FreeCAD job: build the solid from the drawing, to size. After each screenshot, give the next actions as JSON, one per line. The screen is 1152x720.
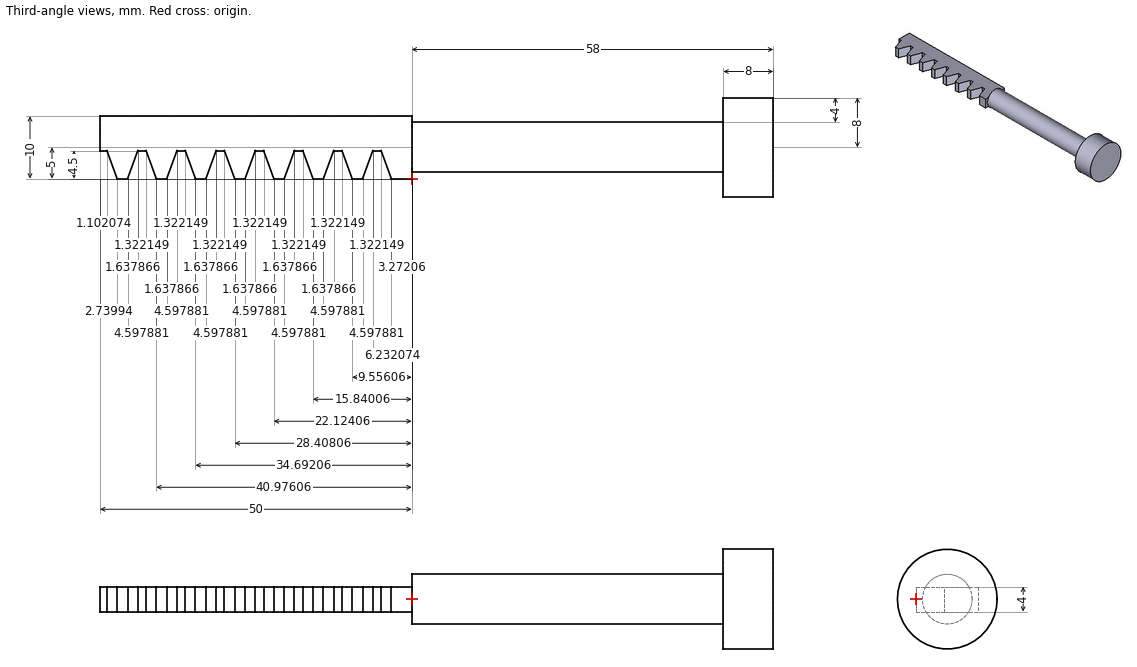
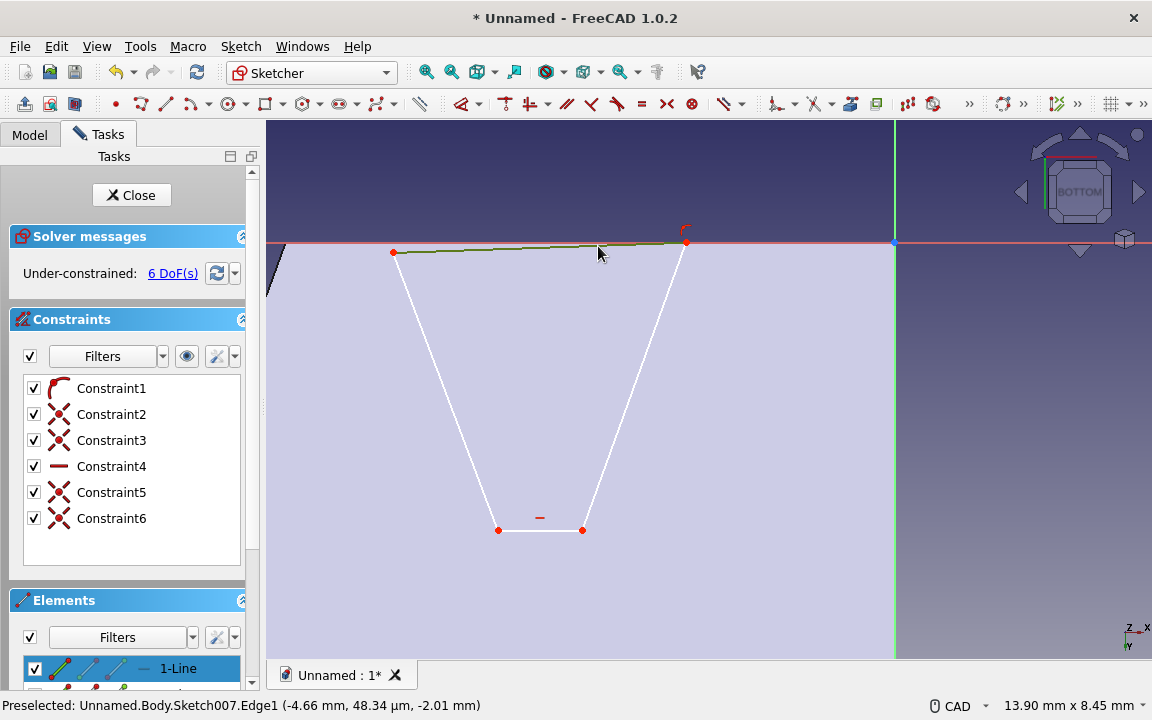
{"action": "key", "text": "h"}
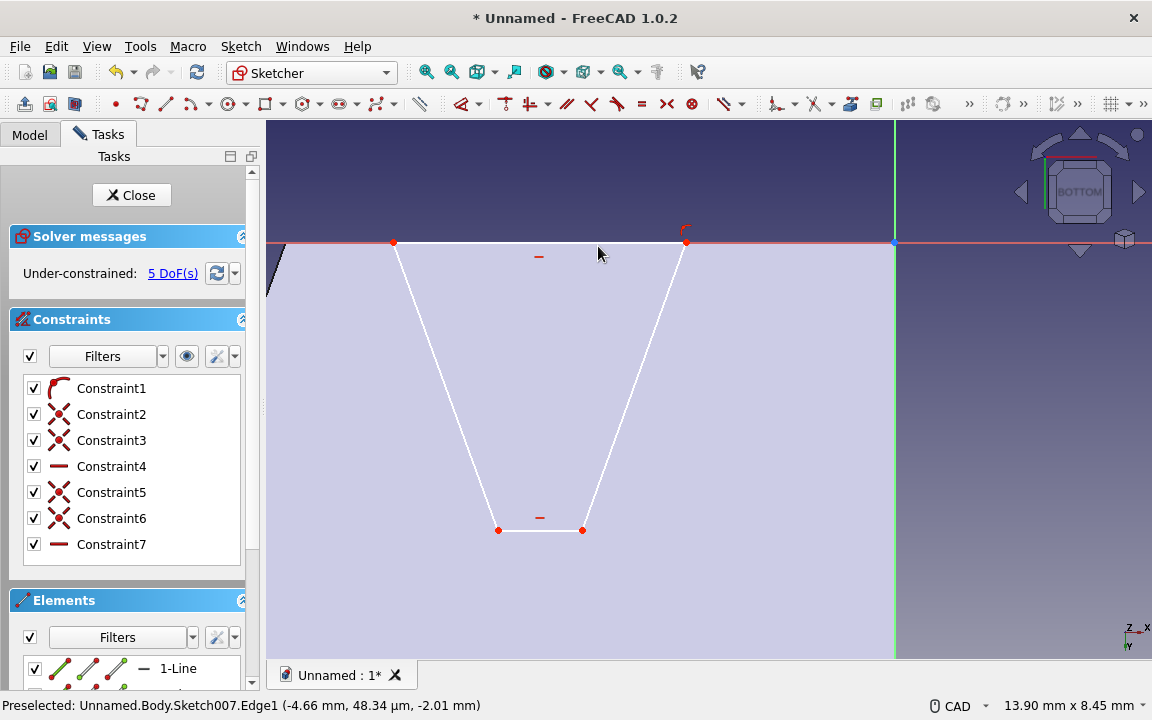
{"action": "left_click", "coordinate": [460, 104]}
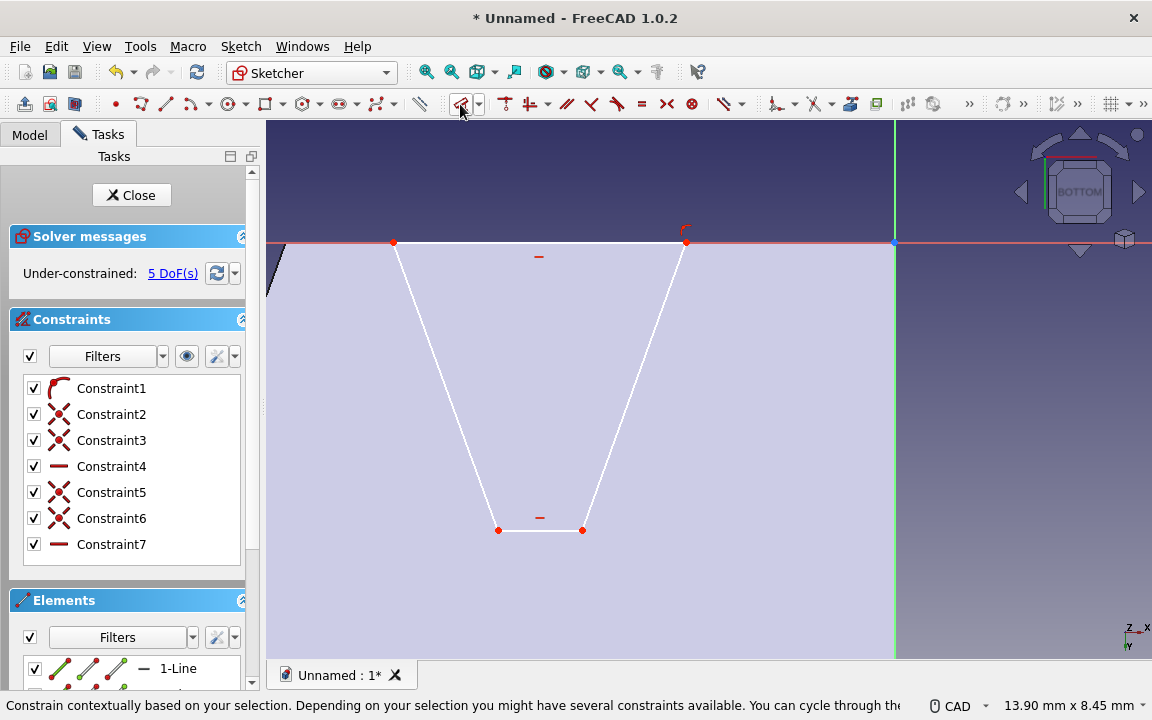
{"action": "left_click", "coordinate": [498, 531]}
{"action": "left_click", "coordinate": [929, 387]}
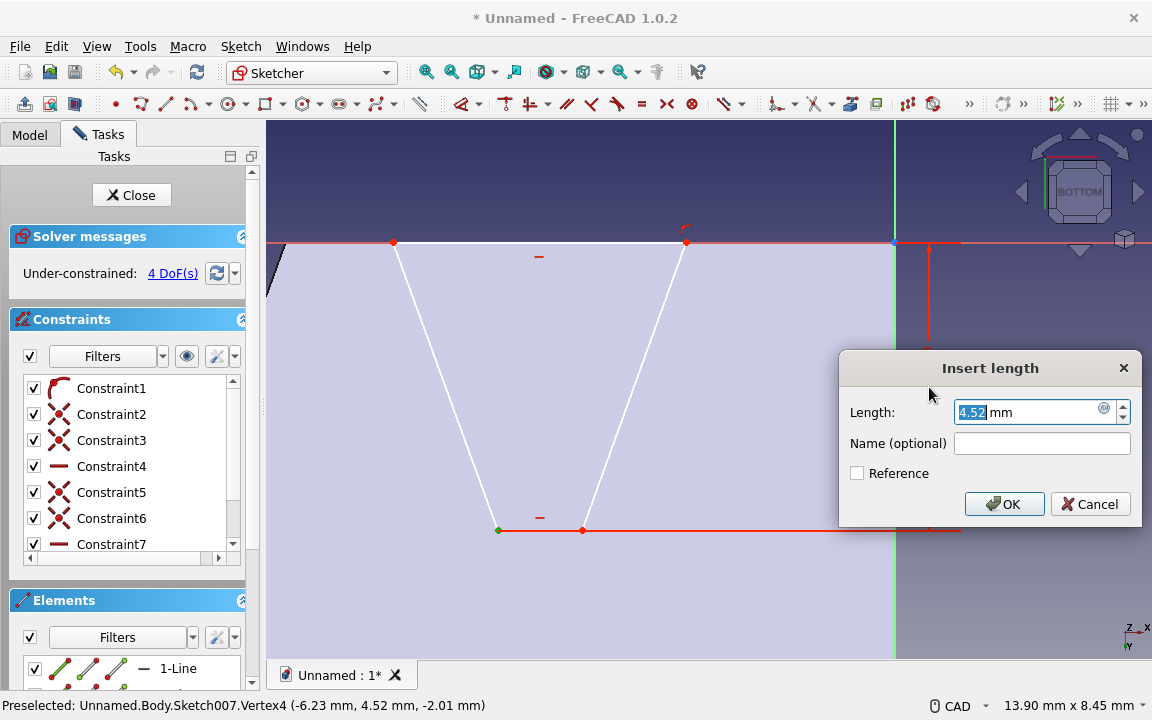
{"action": "type", "text": "4.5"}
{"action": "key", "text": "Return"}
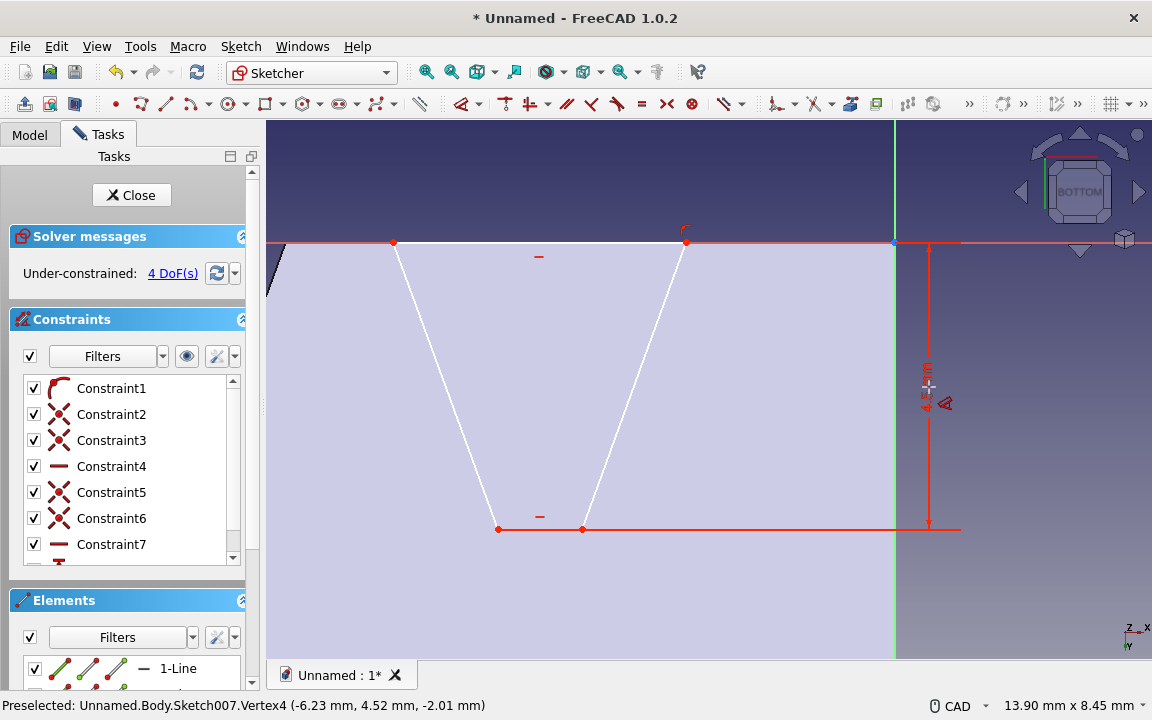
{"action": "left_click", "coordinate": [598, 243]}
{"action": "left_click", "coordinate": [539, 209]}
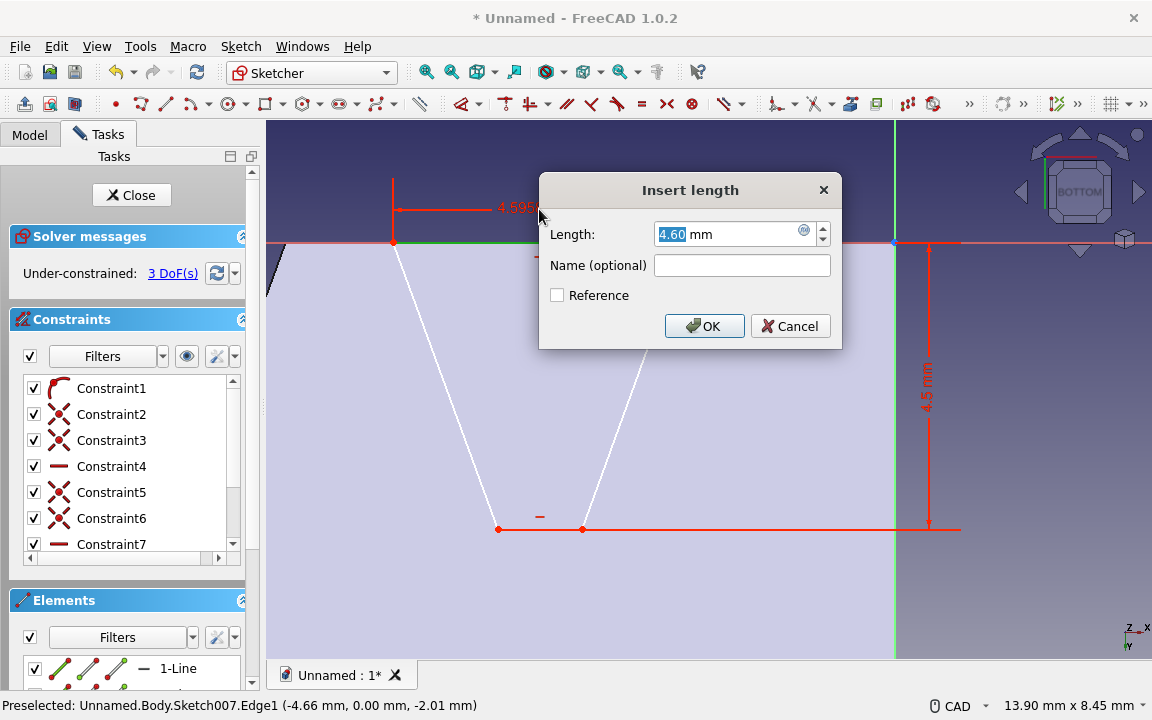
{"action": "type", "text": "4.597881"}
{"action": "key", "text": "Return"}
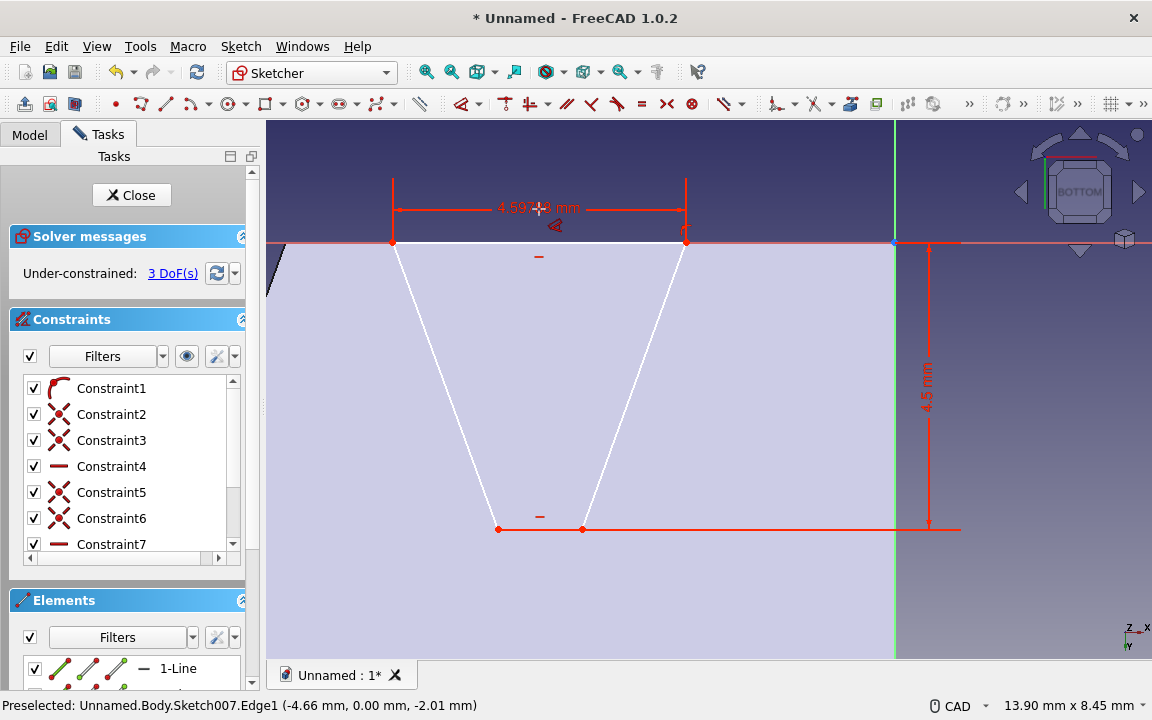
{"action": "left_click", "coordinate": [523, 530]}
{"action": "left_click", "coordinate": [540, 564]}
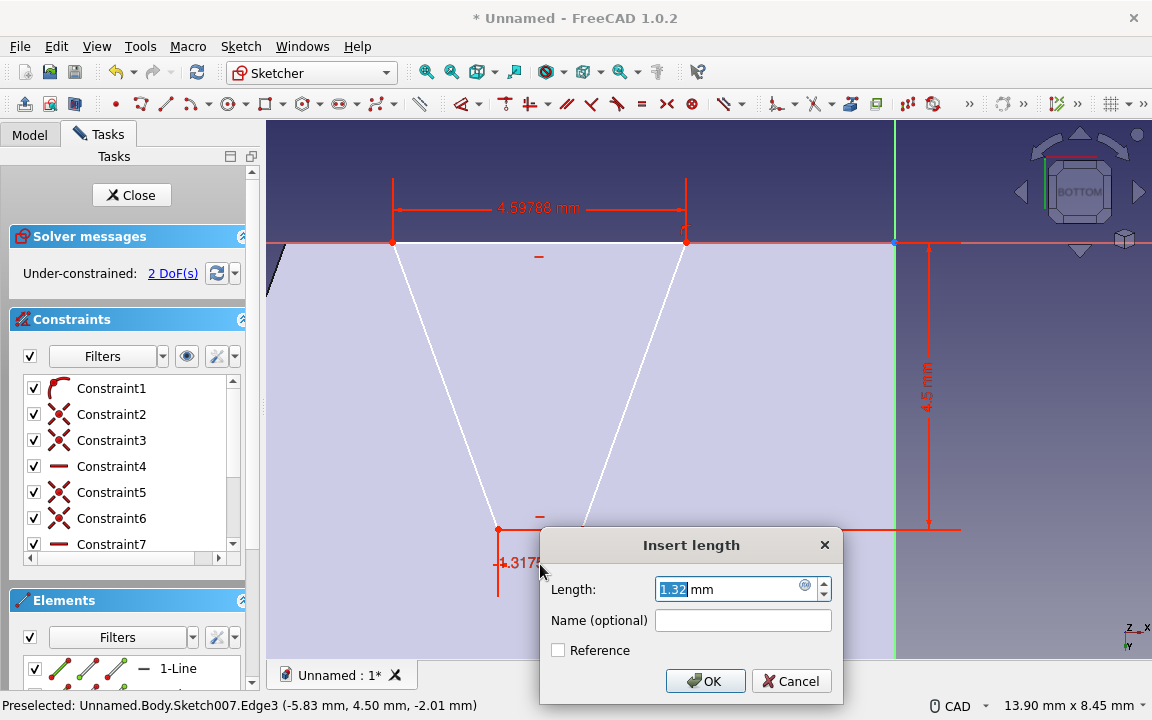
{"action": "type", "text": "1.322149"}
{"action": "key", "text": "Return"}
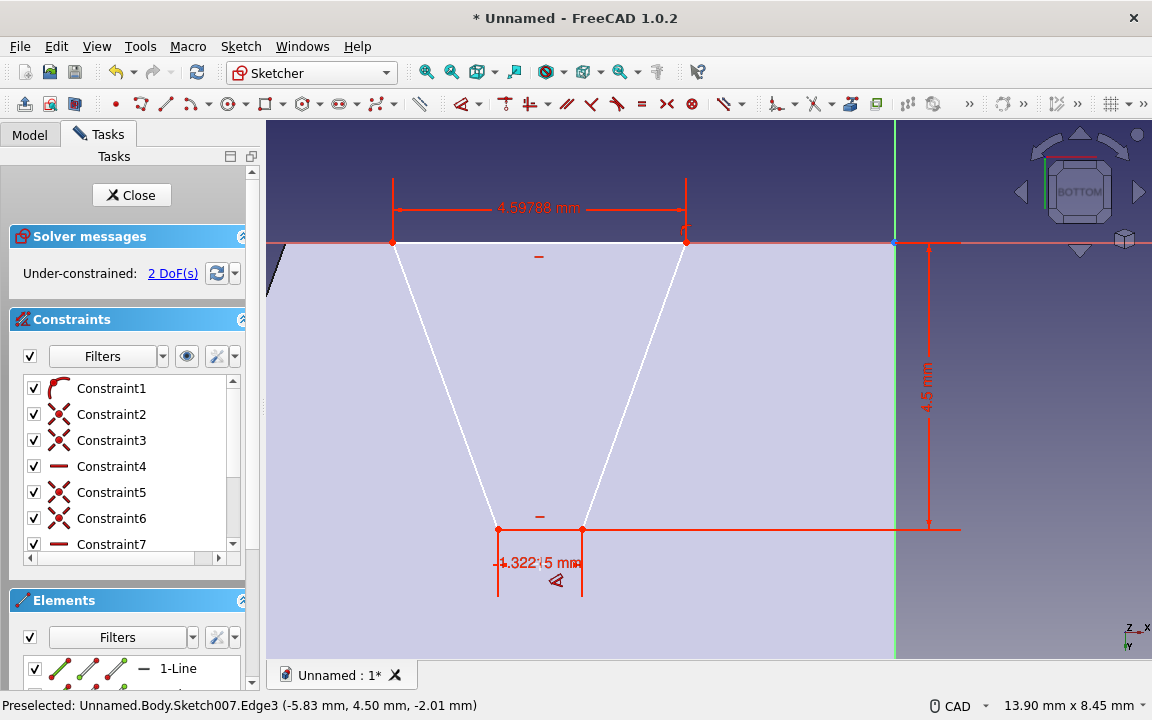
{"action": "left_click", "coordinate": [686, 243]}
{"action": "left_click", "coordinate": [790, 209]}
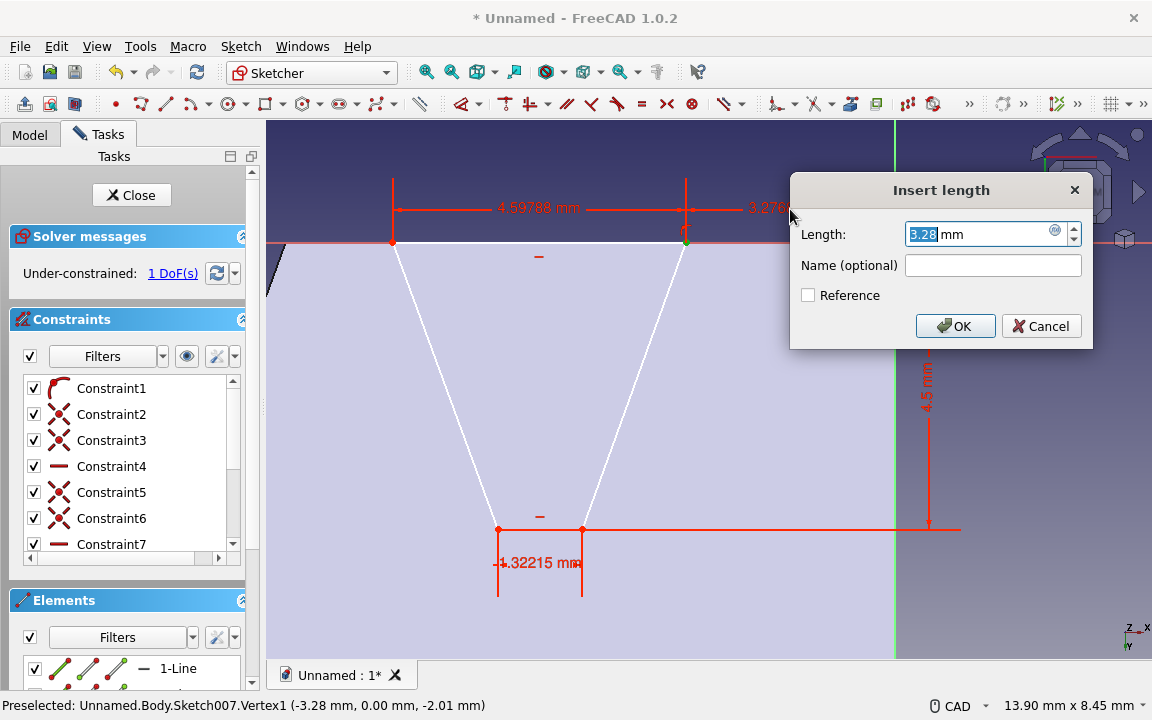
{"action": "type", "text": "3.27206"}
{"action": "key", "text": "Return"}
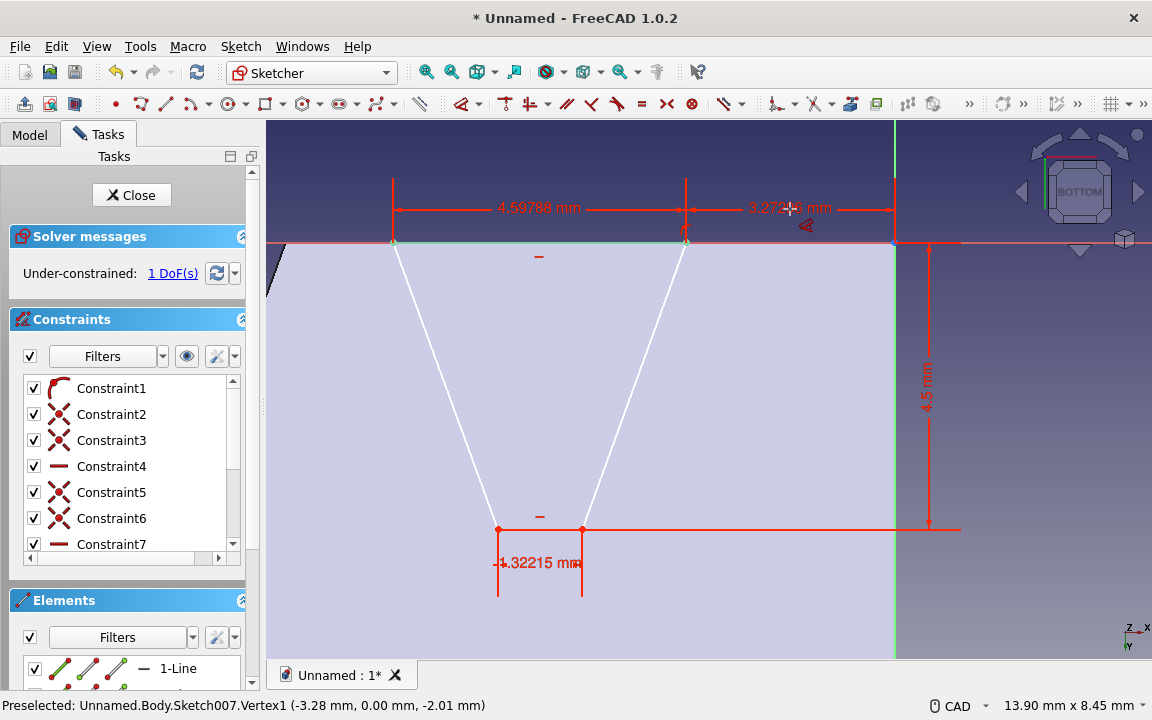
{"action": "left_click", "coordinate": [498, 530]}
{"action": "left_click", "coordinate": [696, 564]}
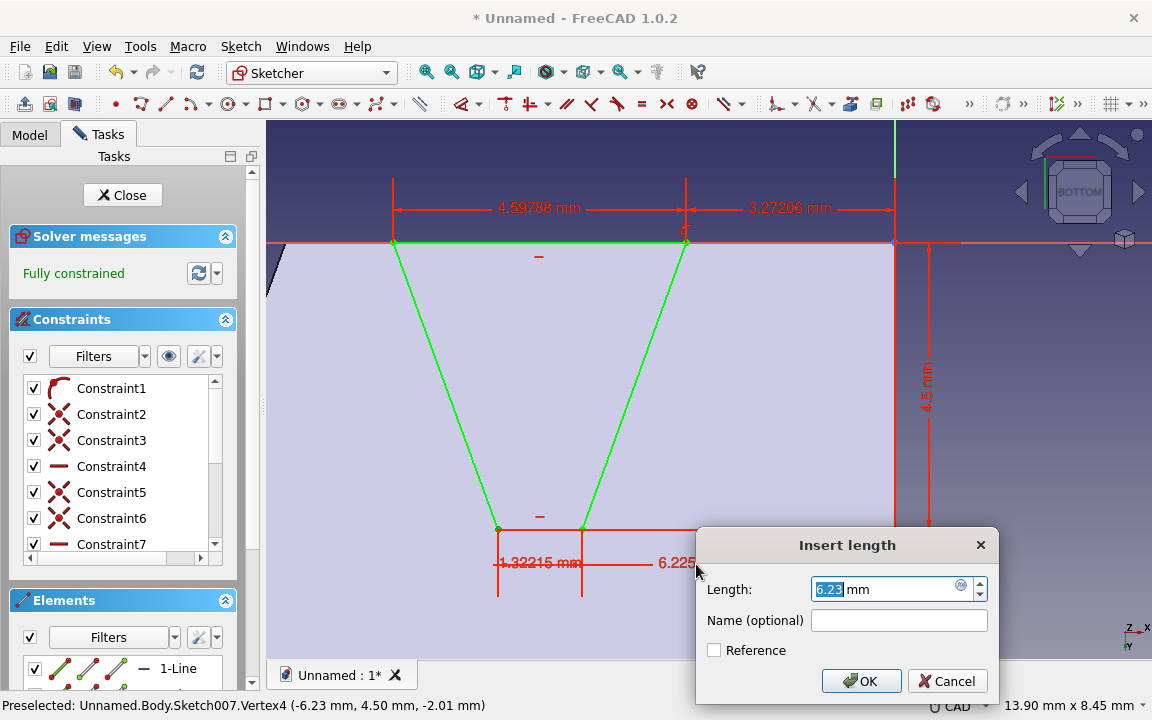
{"action": "type", "text": "6.232074"}
{"action": "key", "text": "Return"}
{"action": "key", "text": "Escape"}